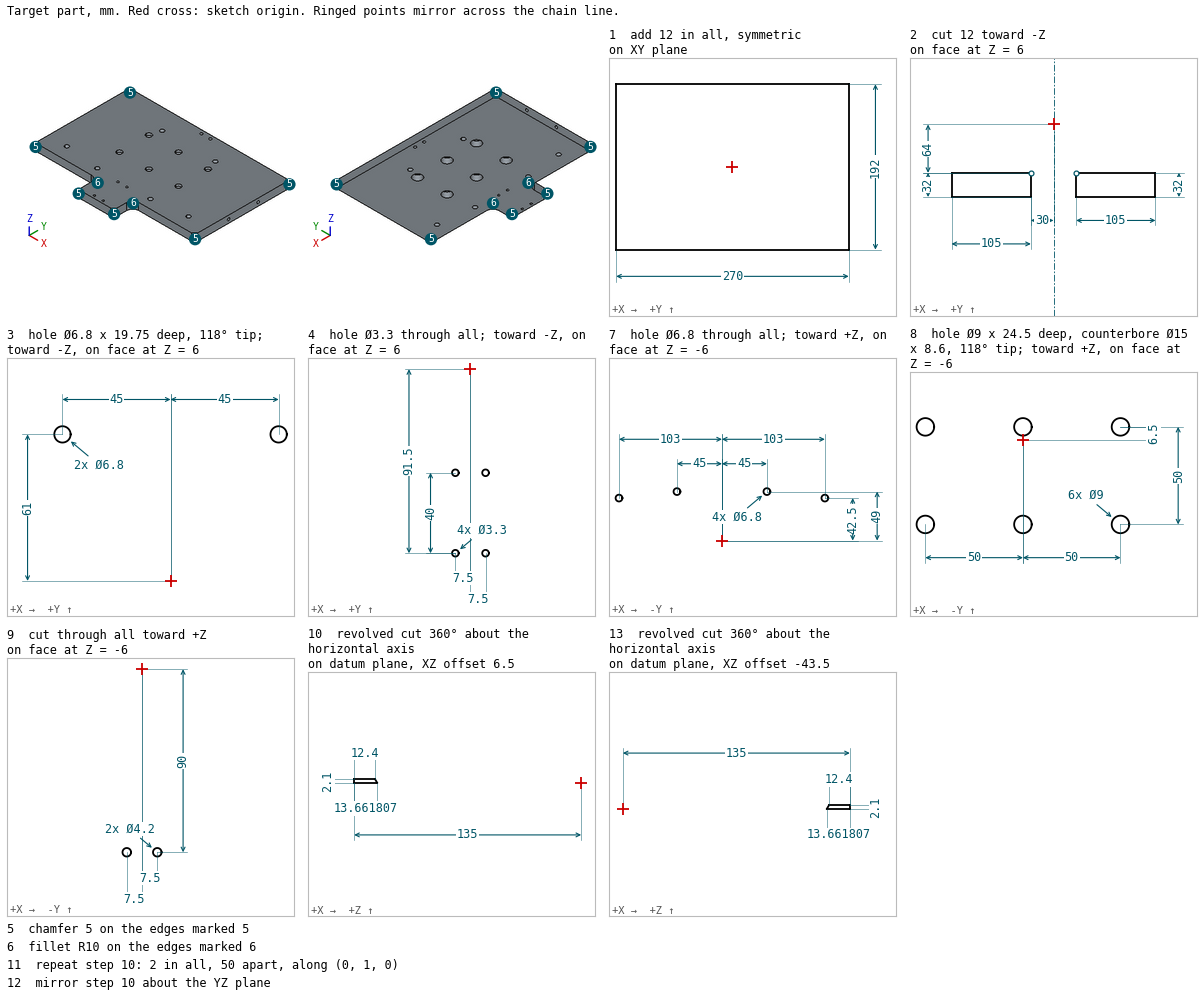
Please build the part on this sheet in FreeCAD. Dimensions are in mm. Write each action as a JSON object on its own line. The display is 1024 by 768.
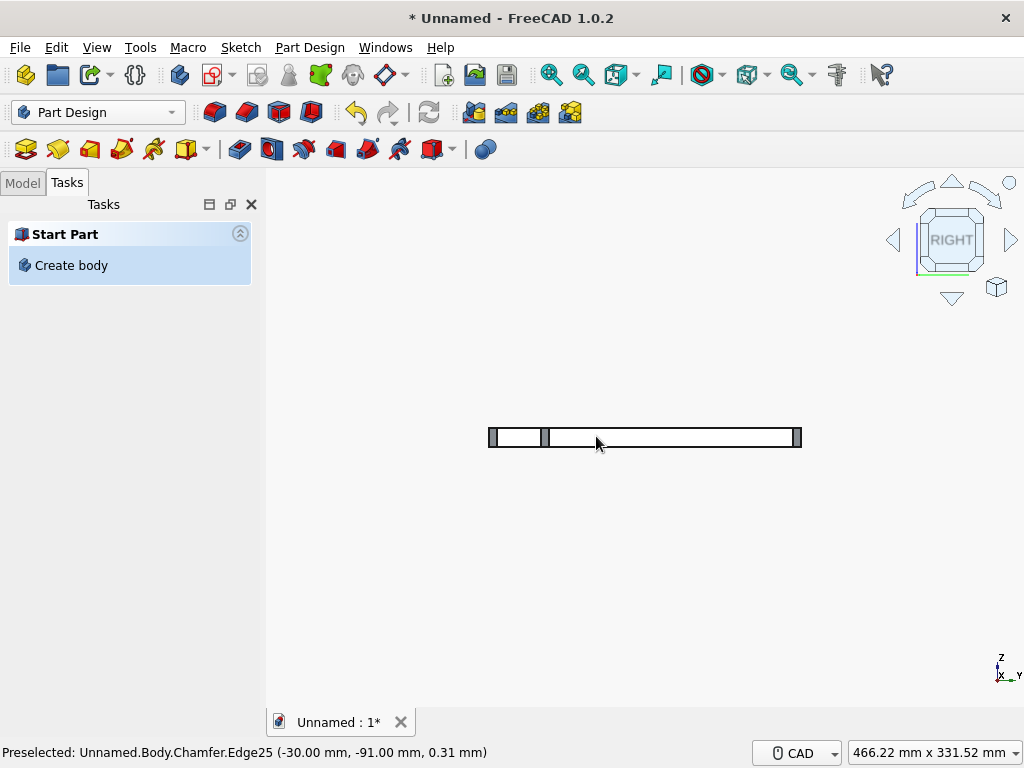
{"action": "scroll", "coordinate": [541, 436], "scroll_direction": "up", "scroll_amount": 4}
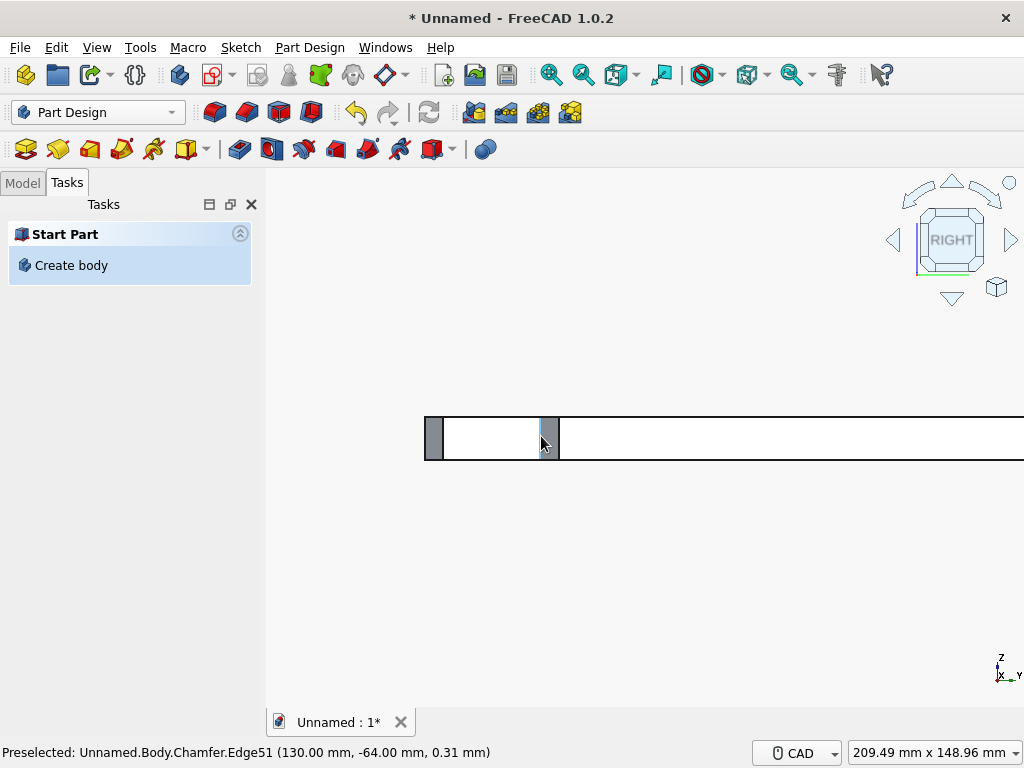
{"action": "left_click", "coordinate": [552, 76]}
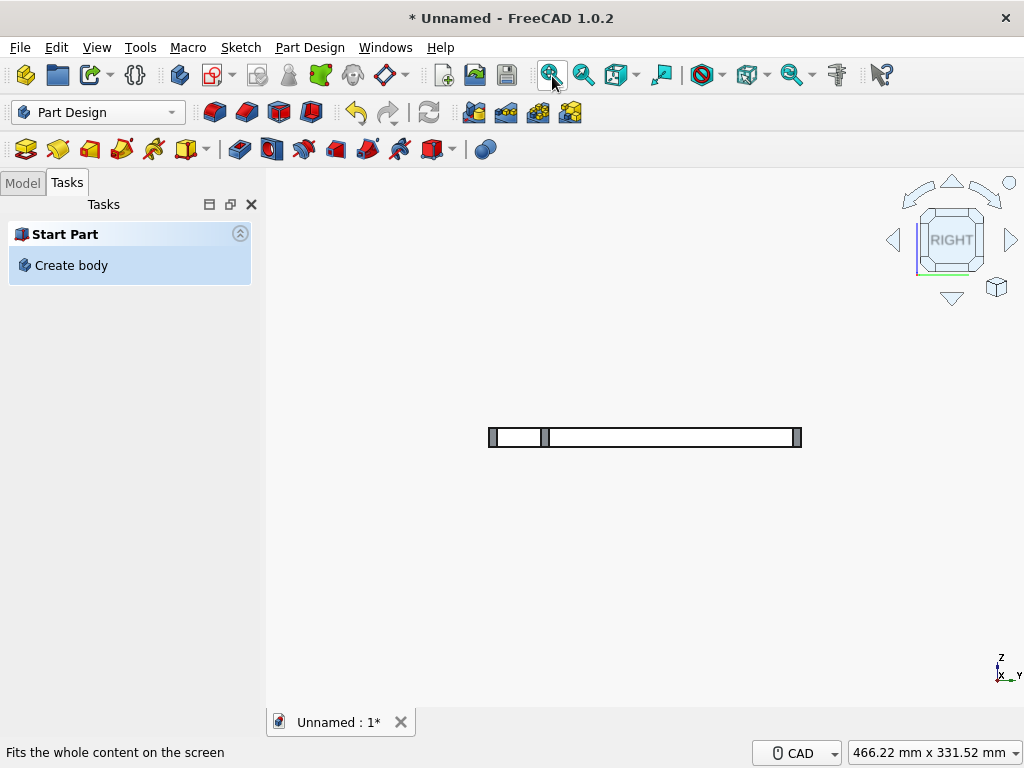
{"action": "key", "text": "5"}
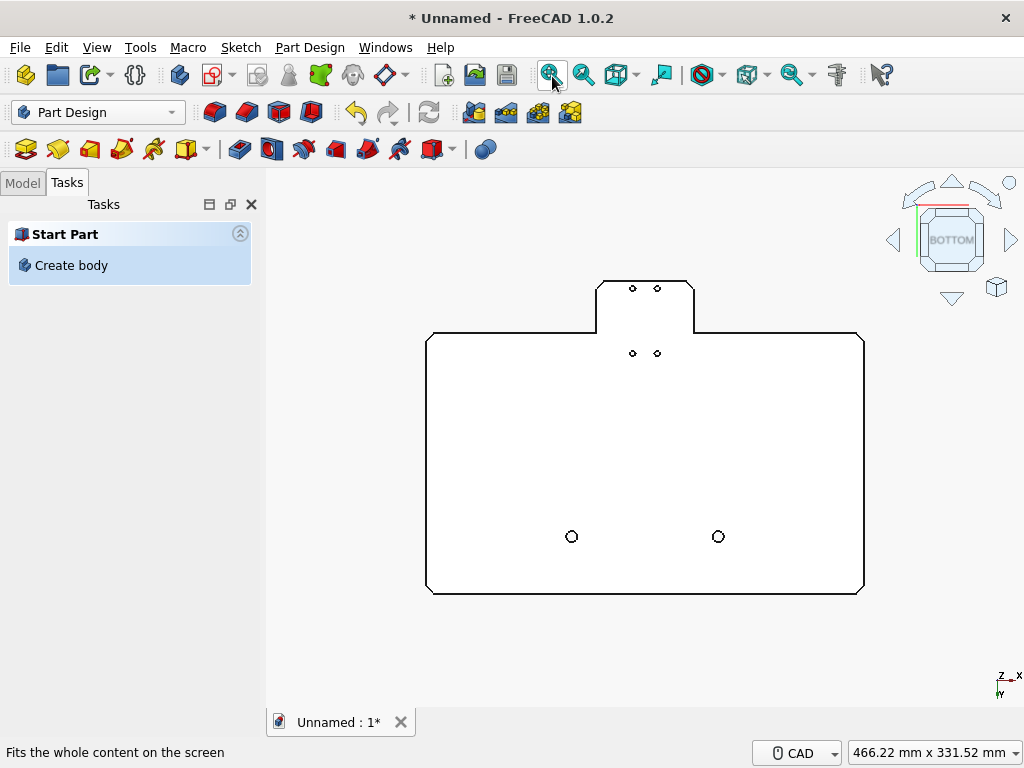
{"action": "scroll", "coordinate": [596, 332], "scroll_direction": "up", "scroll_amount": 4}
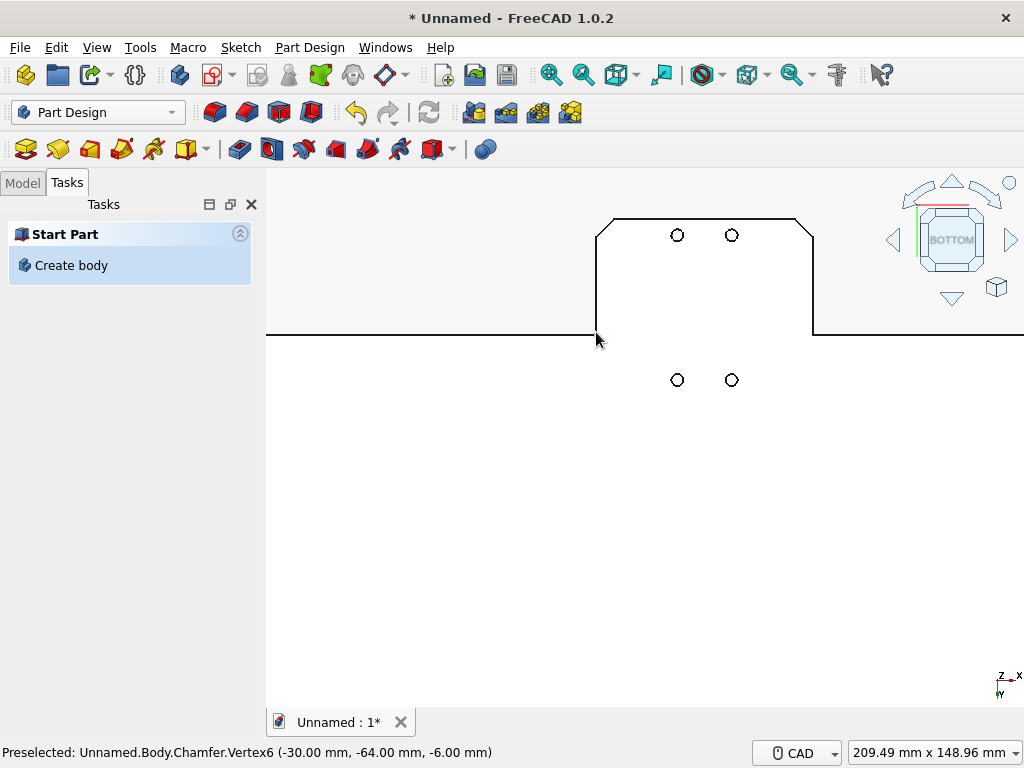
{"action": "key", "text": "v f"}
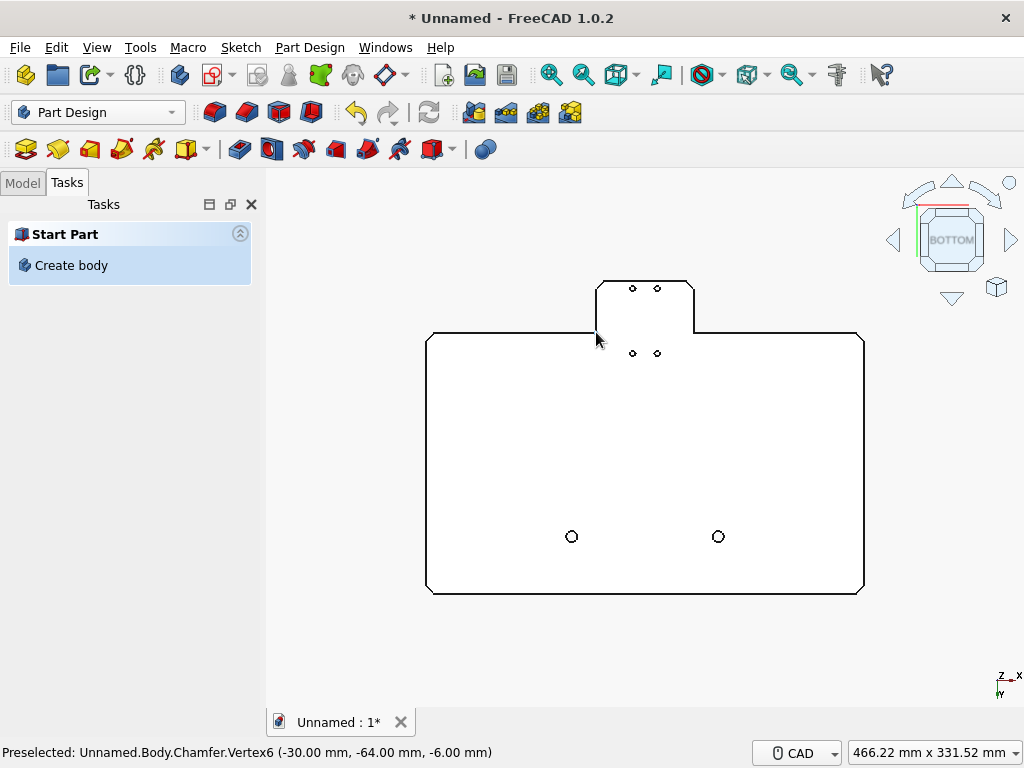
{"action": "key", "text": "4"}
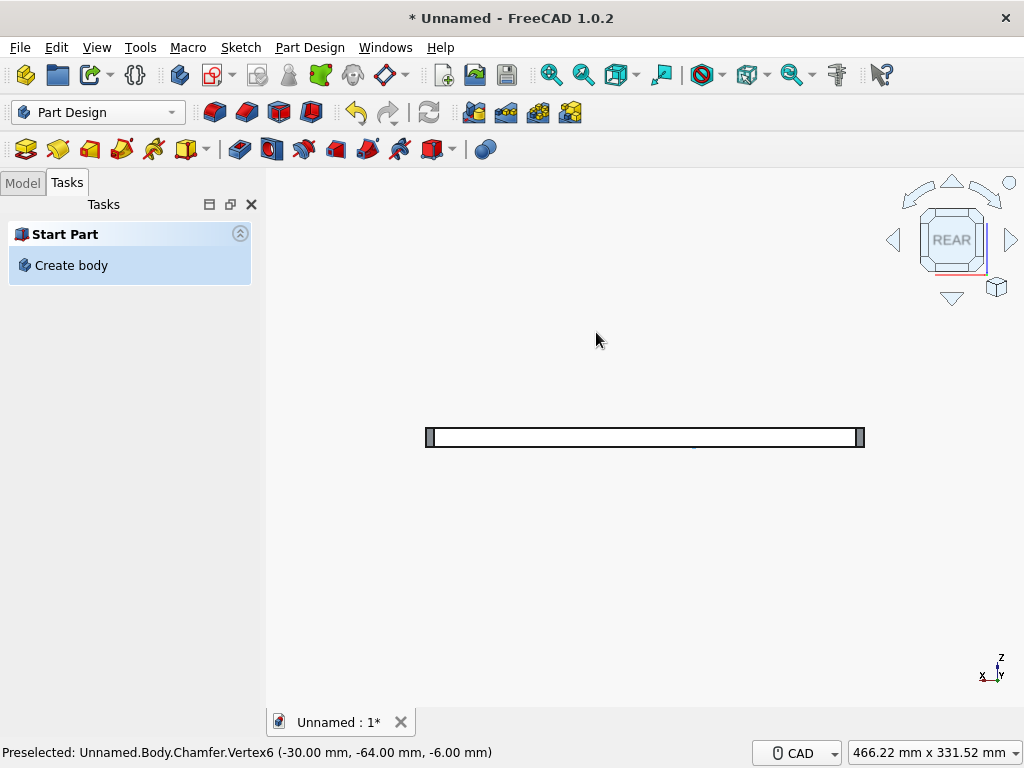
{"action": "scroll", "coordinate": [694, 436], "scroll_direction": "up", "scroll_amount": 4}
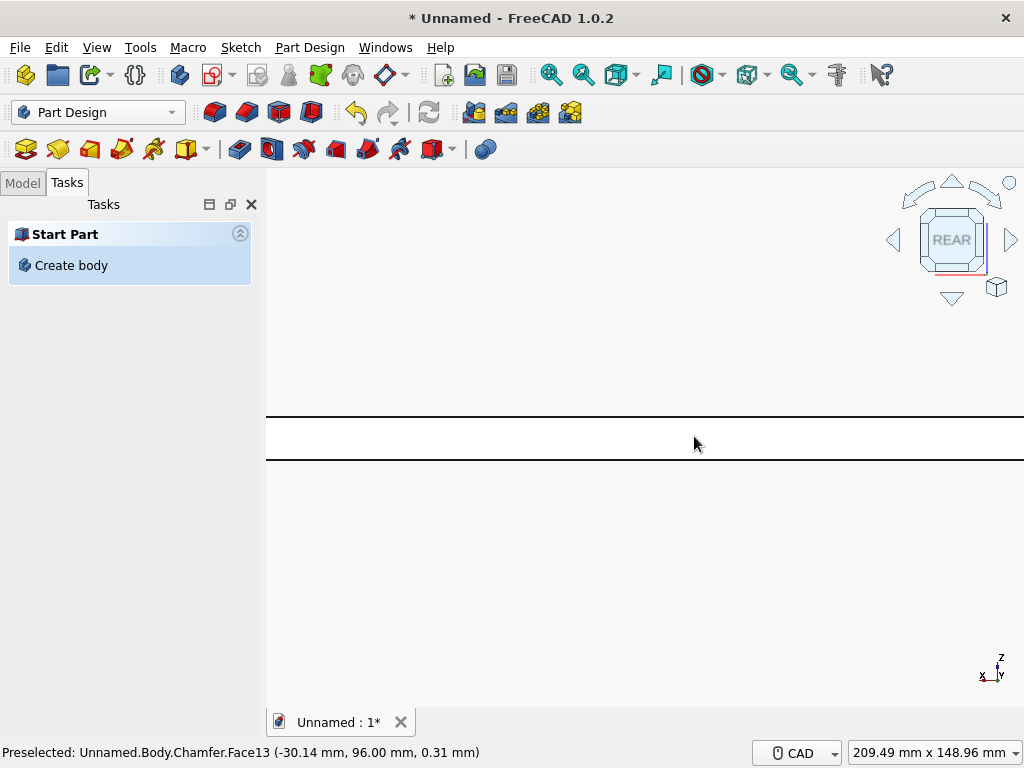
{"action": "key", "text": "v f"}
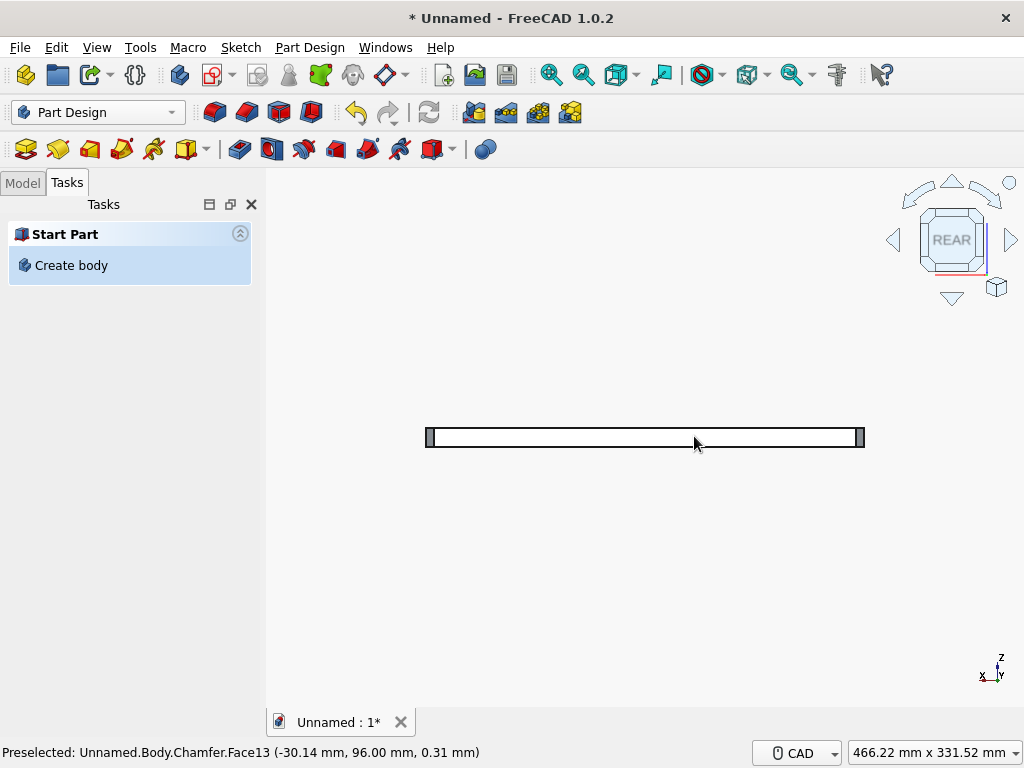
{"action": "key", "text": "6"}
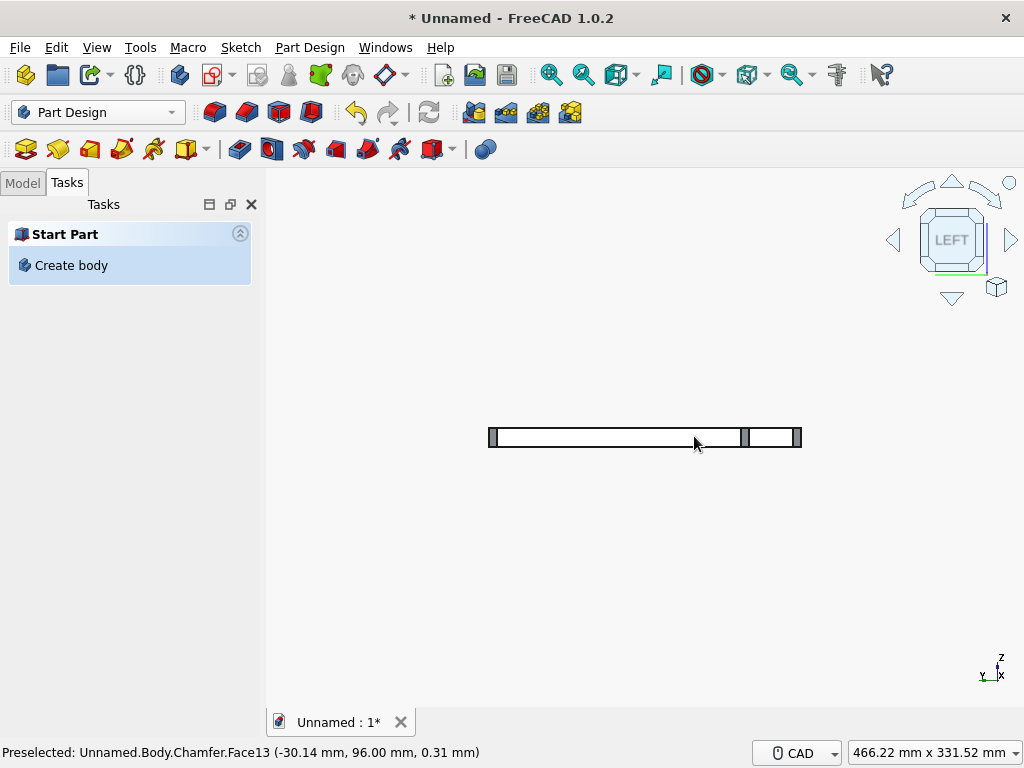
{"action": "key", "text": "v f"}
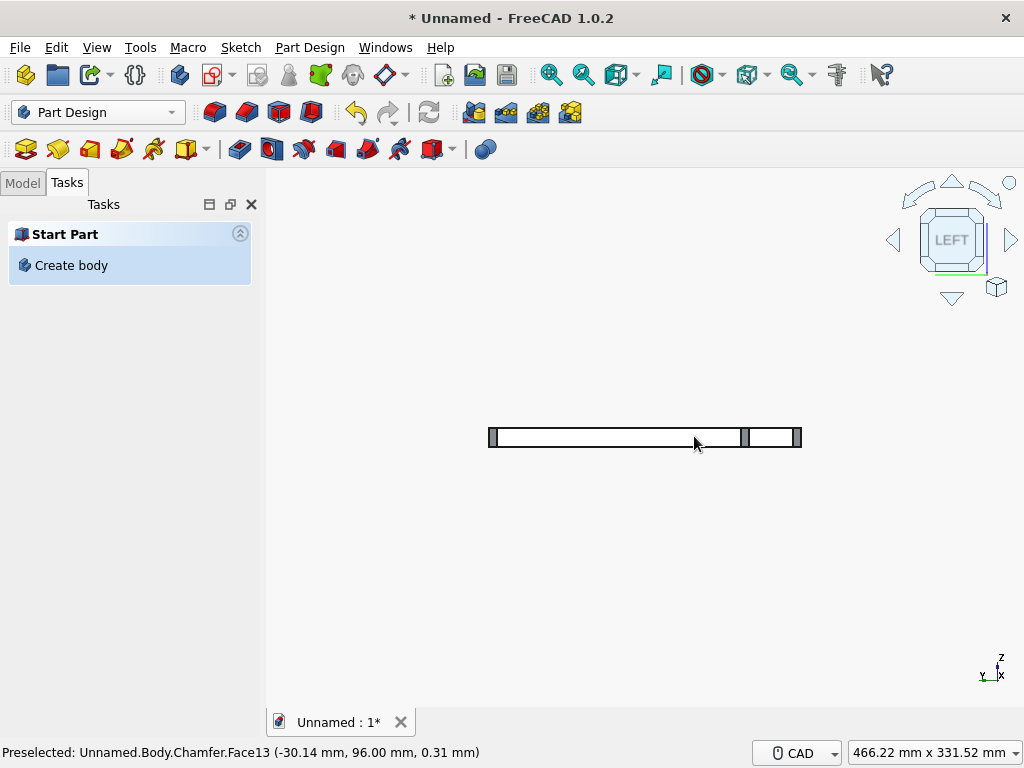
{"action": "scroll", "coordinate": [749, 436], "scroll_direction": "up", "scroll_amount": 4}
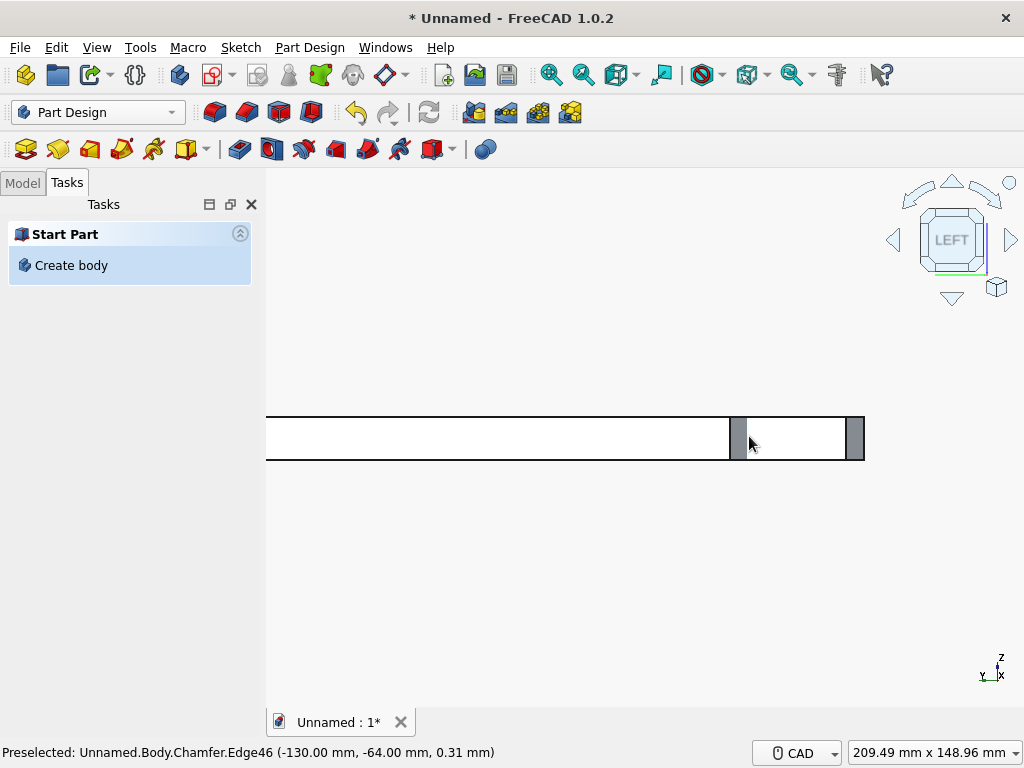
{"action": "key", "text": "v f"}